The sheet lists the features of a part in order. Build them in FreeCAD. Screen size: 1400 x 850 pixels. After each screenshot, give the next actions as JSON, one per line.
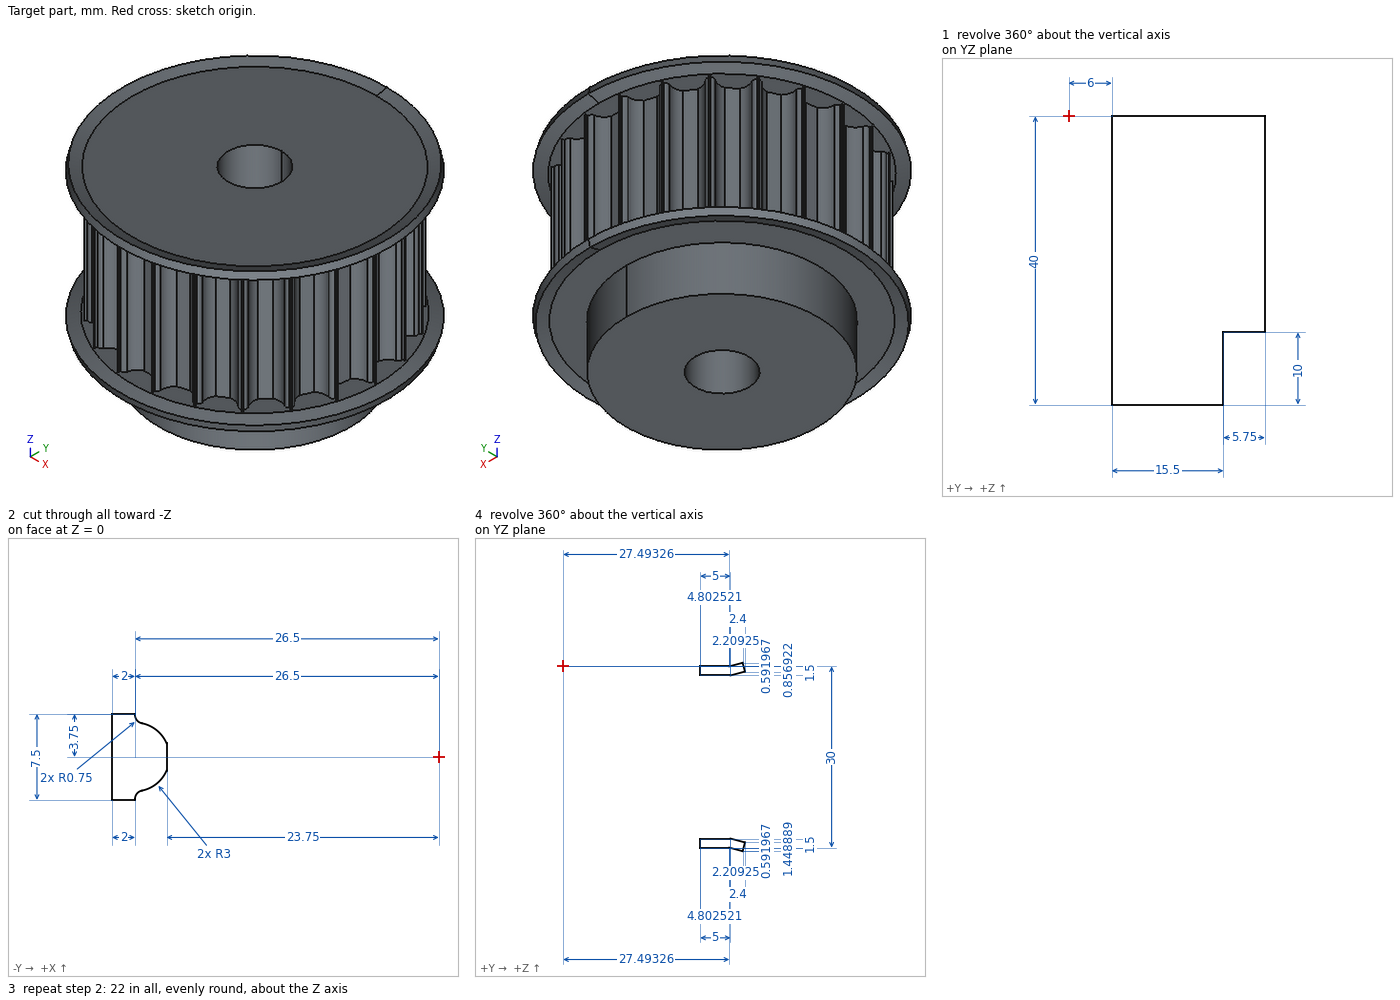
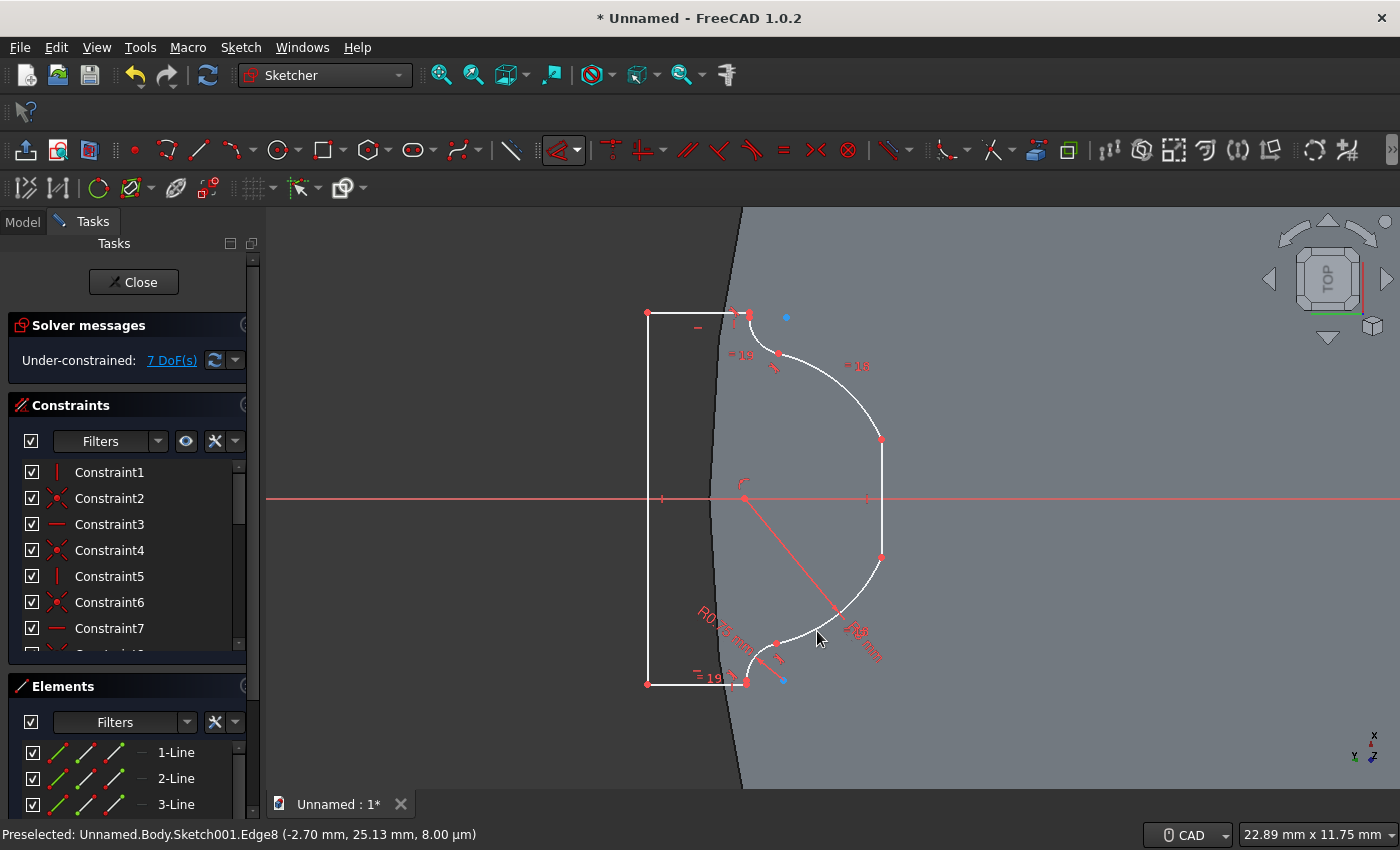
{"action": "left_click", "coordinate": [719, 313]}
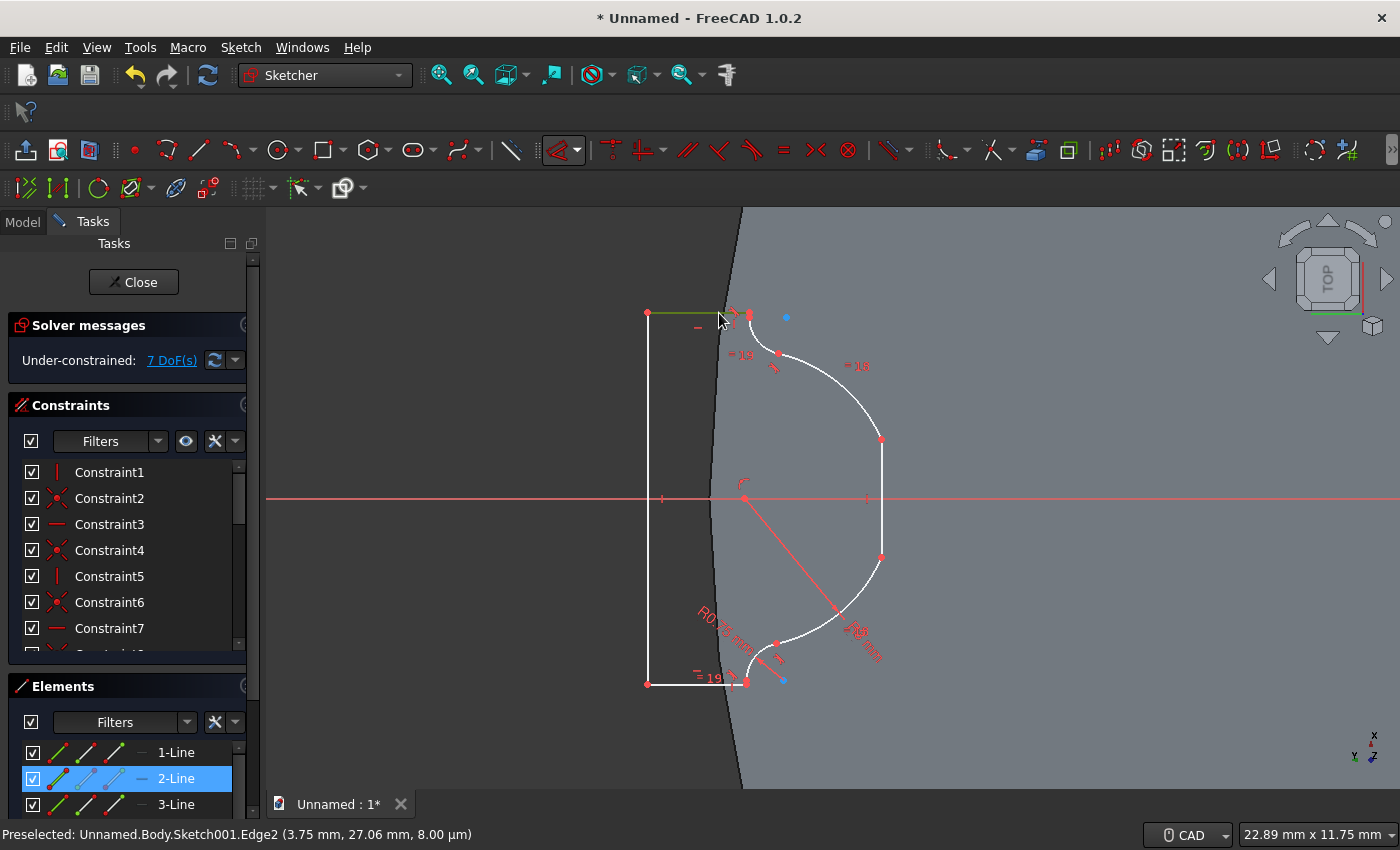
{"action": "left_click", "coordinate": [580, 150]}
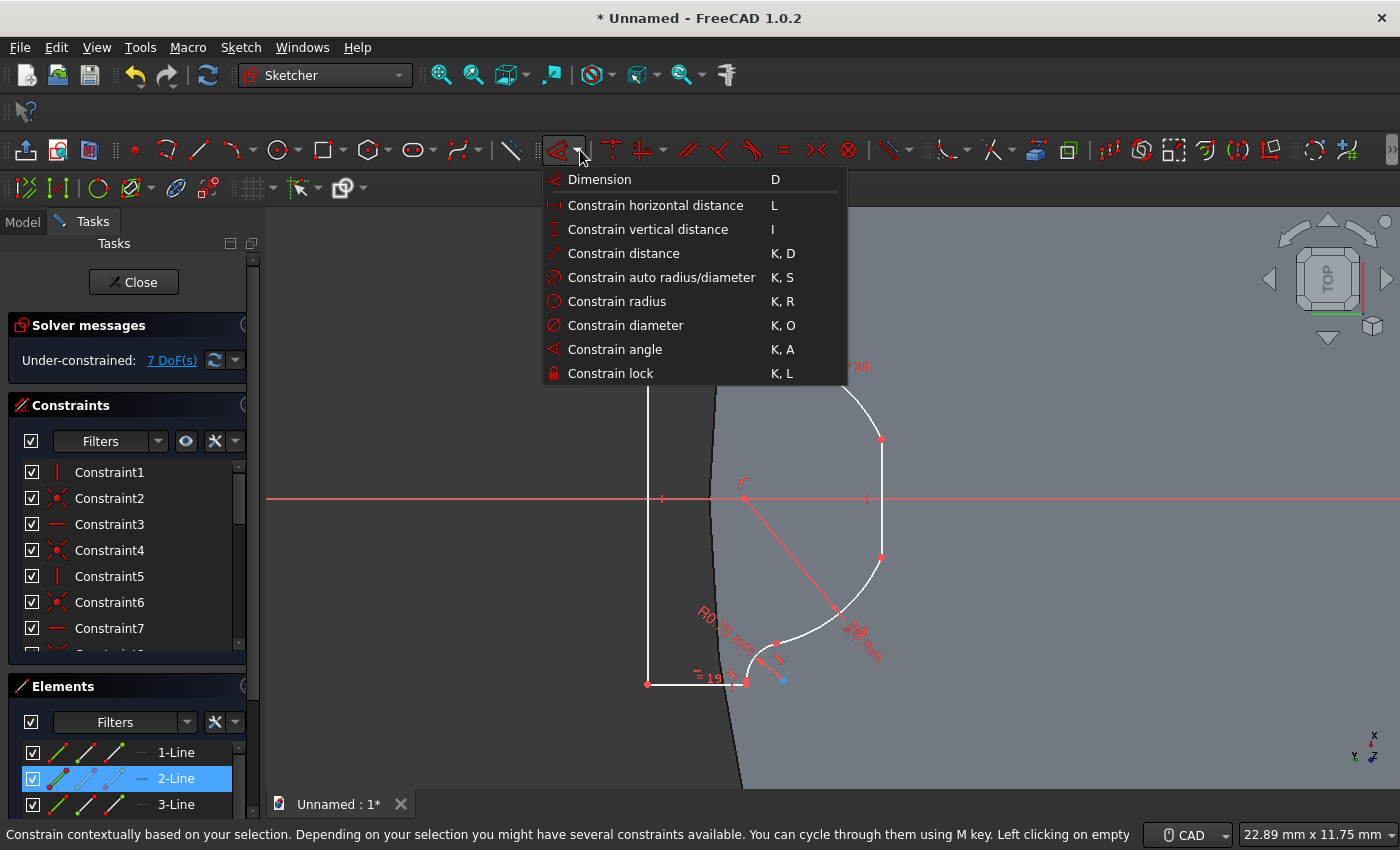
{"action": "left_click", "coordinate": [695, 205]}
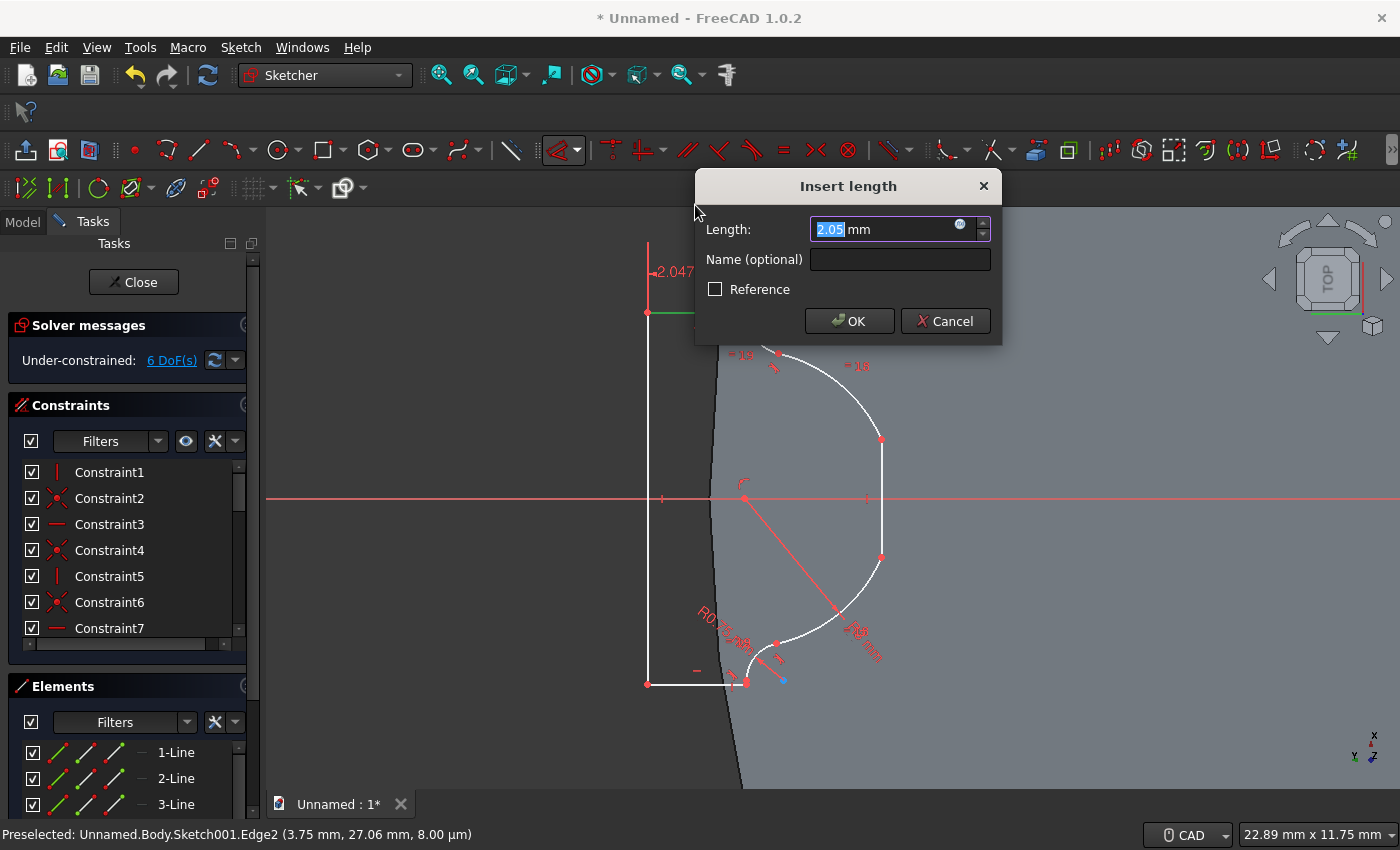
{"action": "type", "text": "2"}
{"action": "key", "text": "Return"}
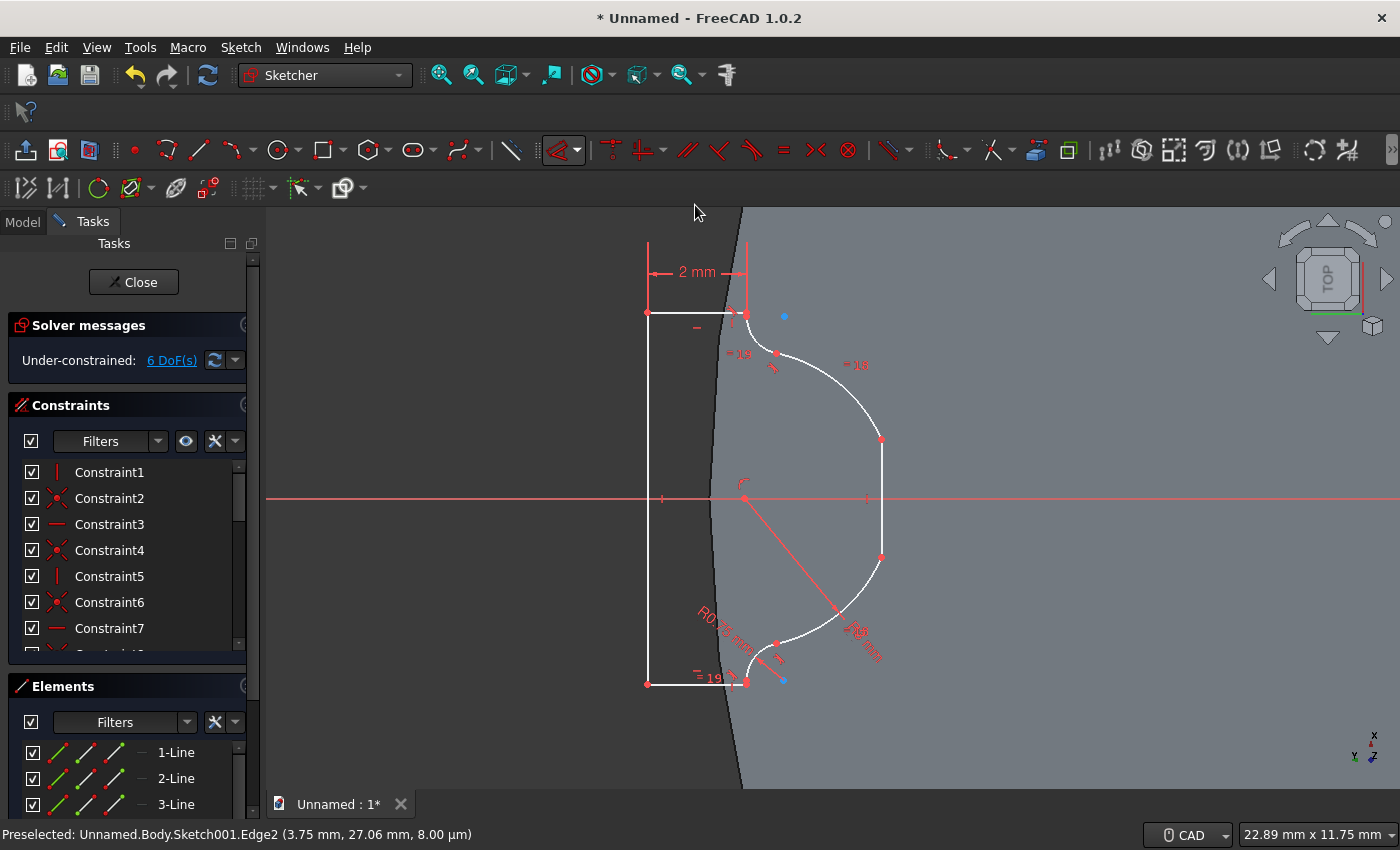
{"action": "left_click", "coordinate": [678, 685]}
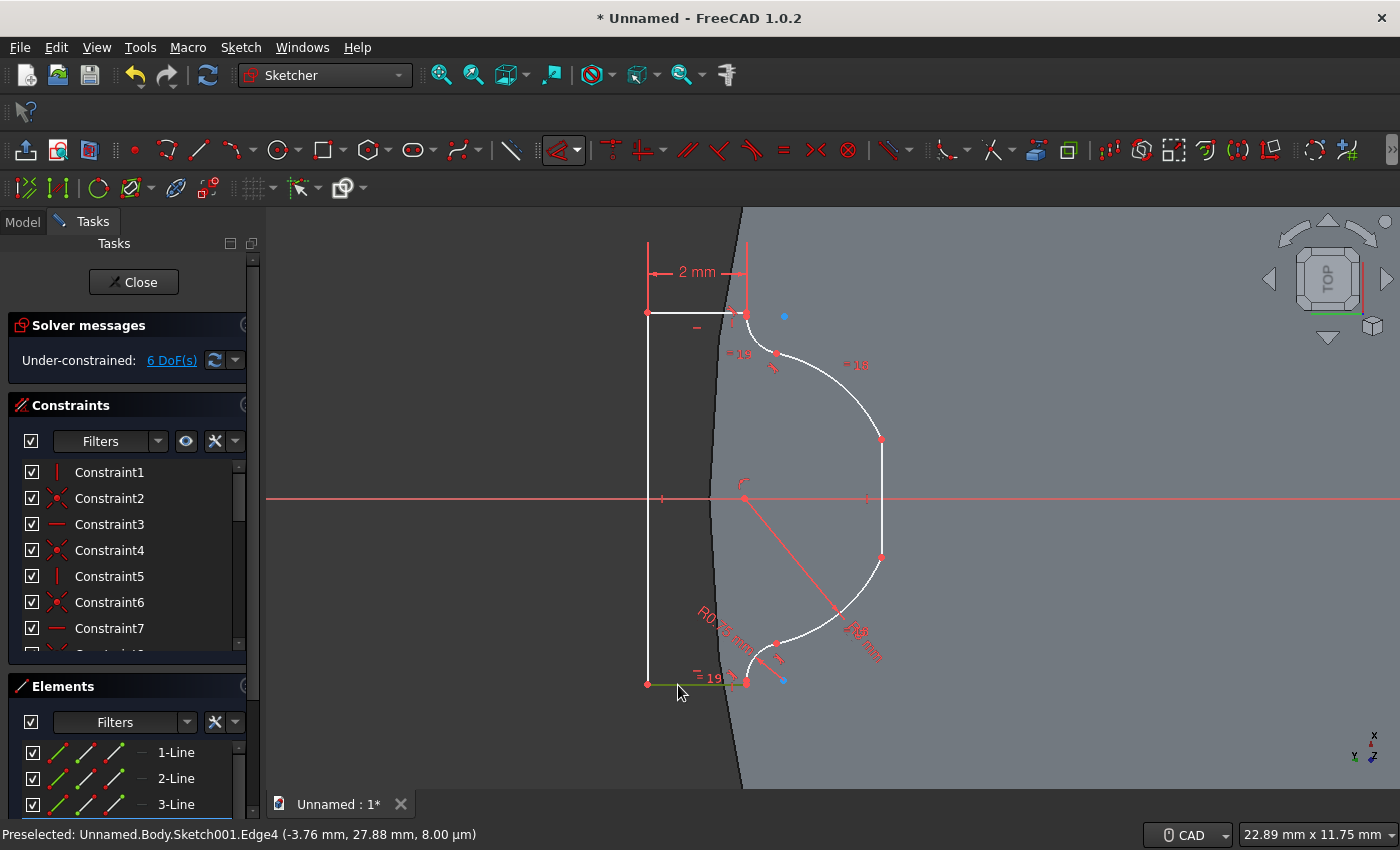
{"action": "left_click", "coordinate": [580, 150]}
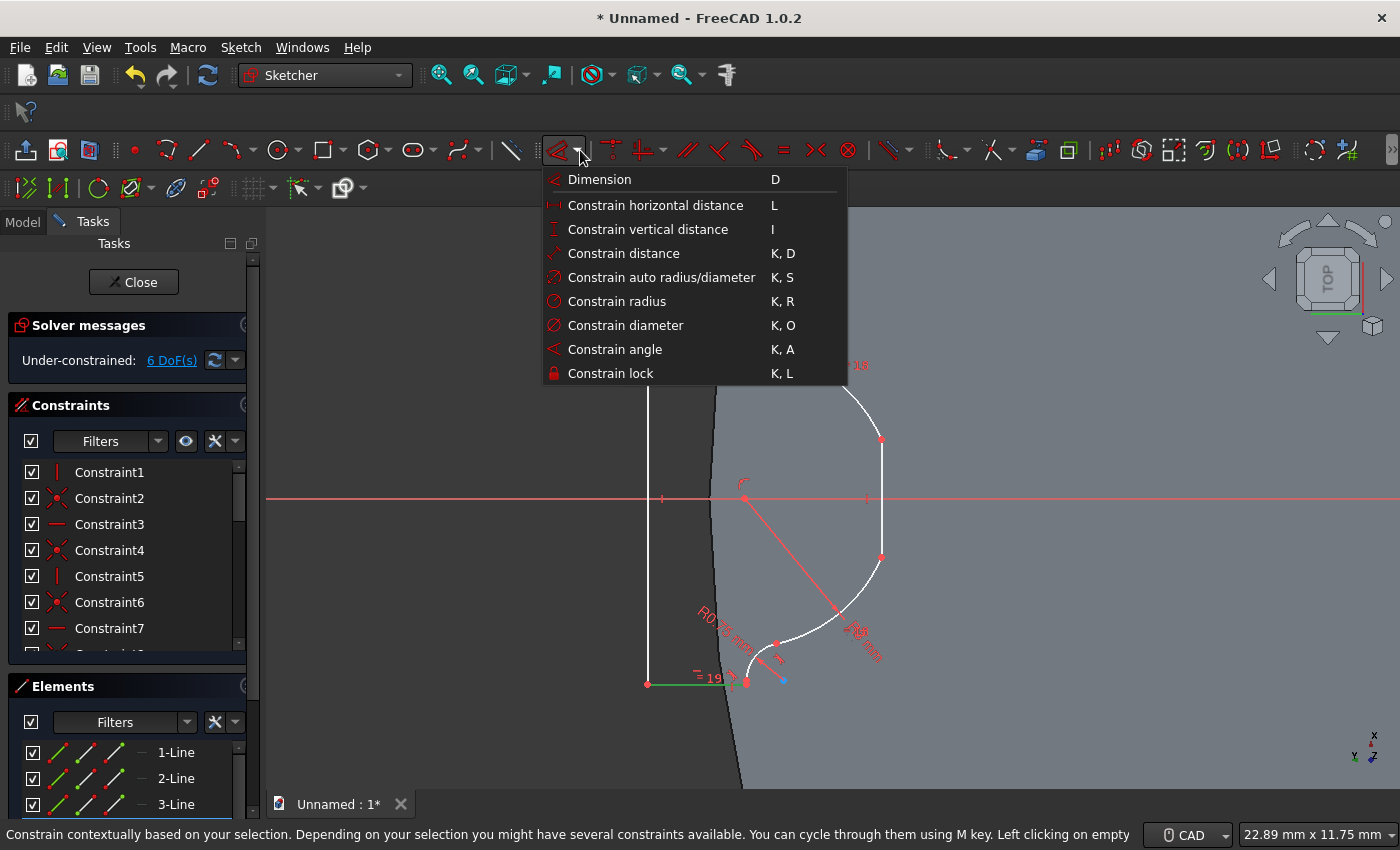
{"action": "left_click", "coordinate": [695, 205]}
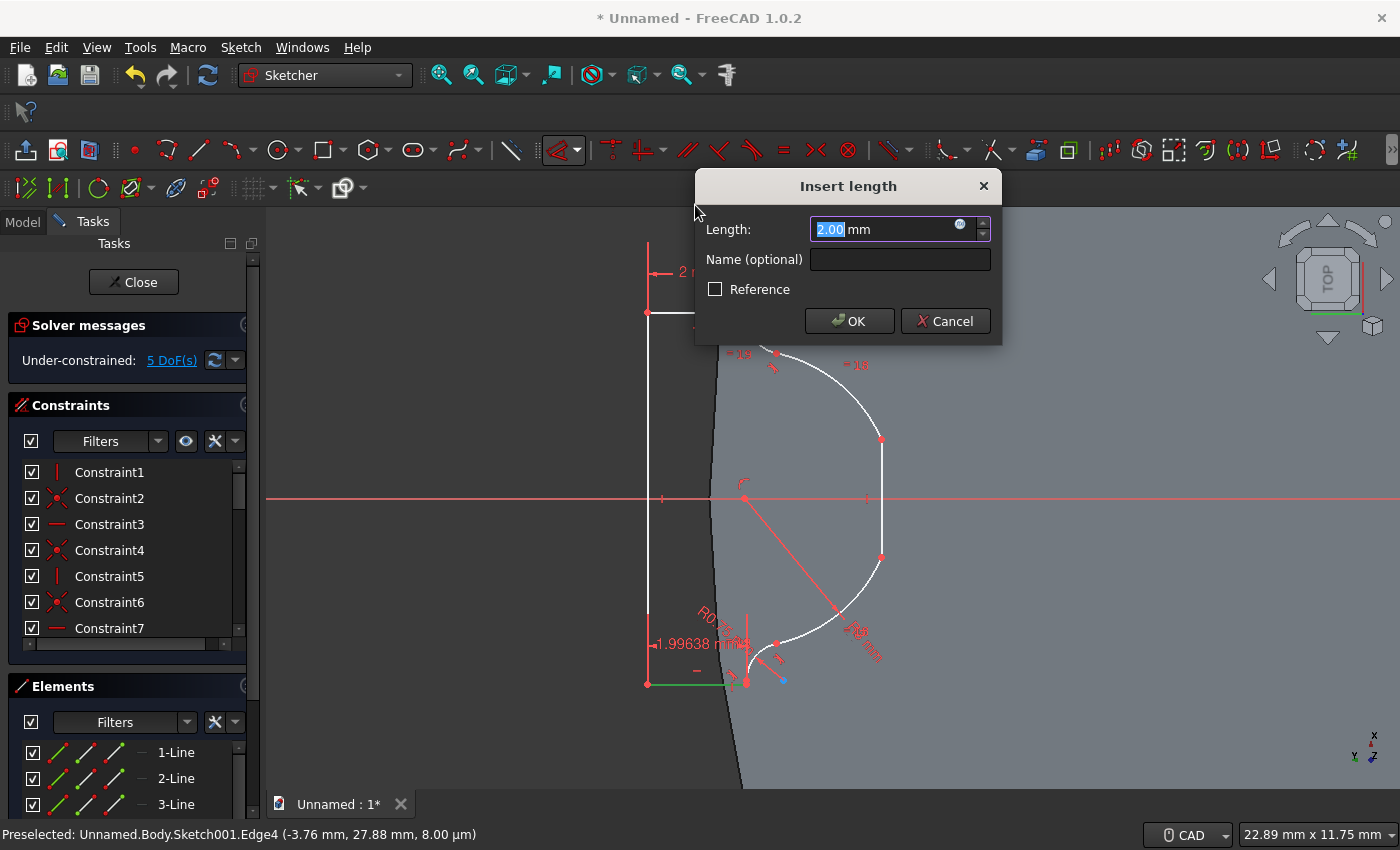
{"action": "type", "text": "2"}
{"action": "key", "text": "Return"}